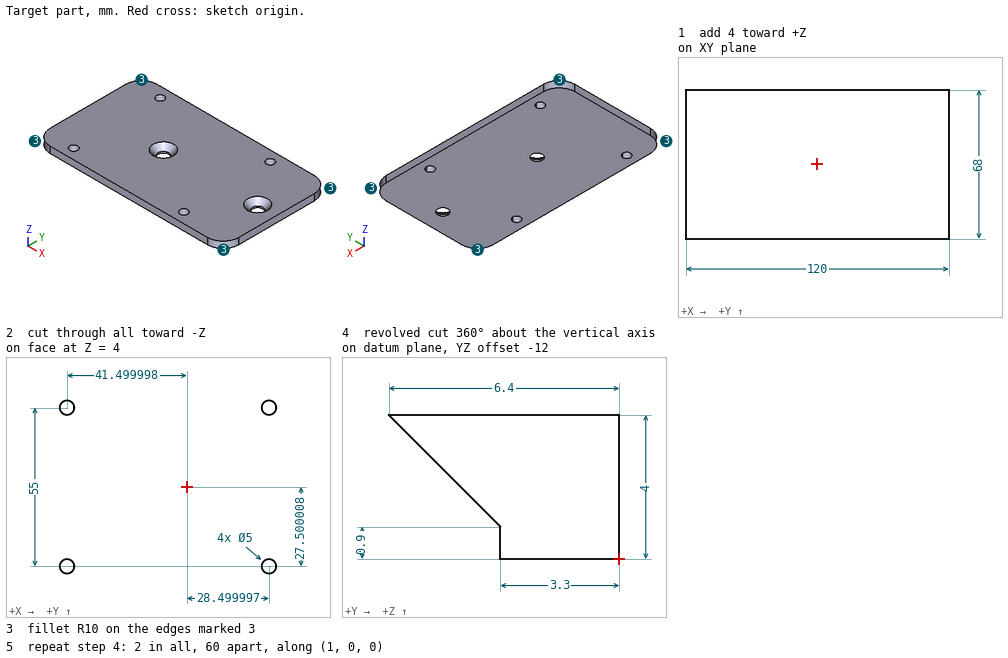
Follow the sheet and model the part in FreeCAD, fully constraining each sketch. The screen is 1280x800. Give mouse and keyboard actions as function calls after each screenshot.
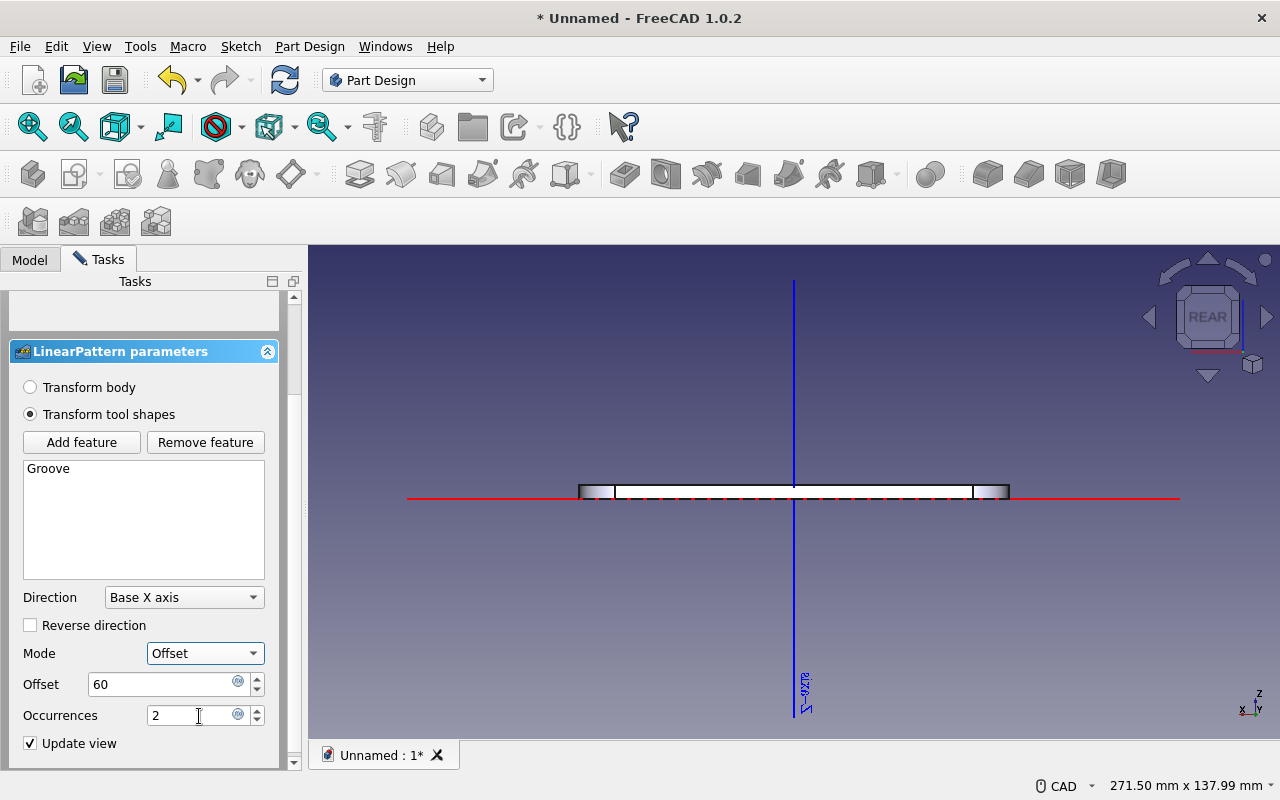
scroll(294, 530, up, 3)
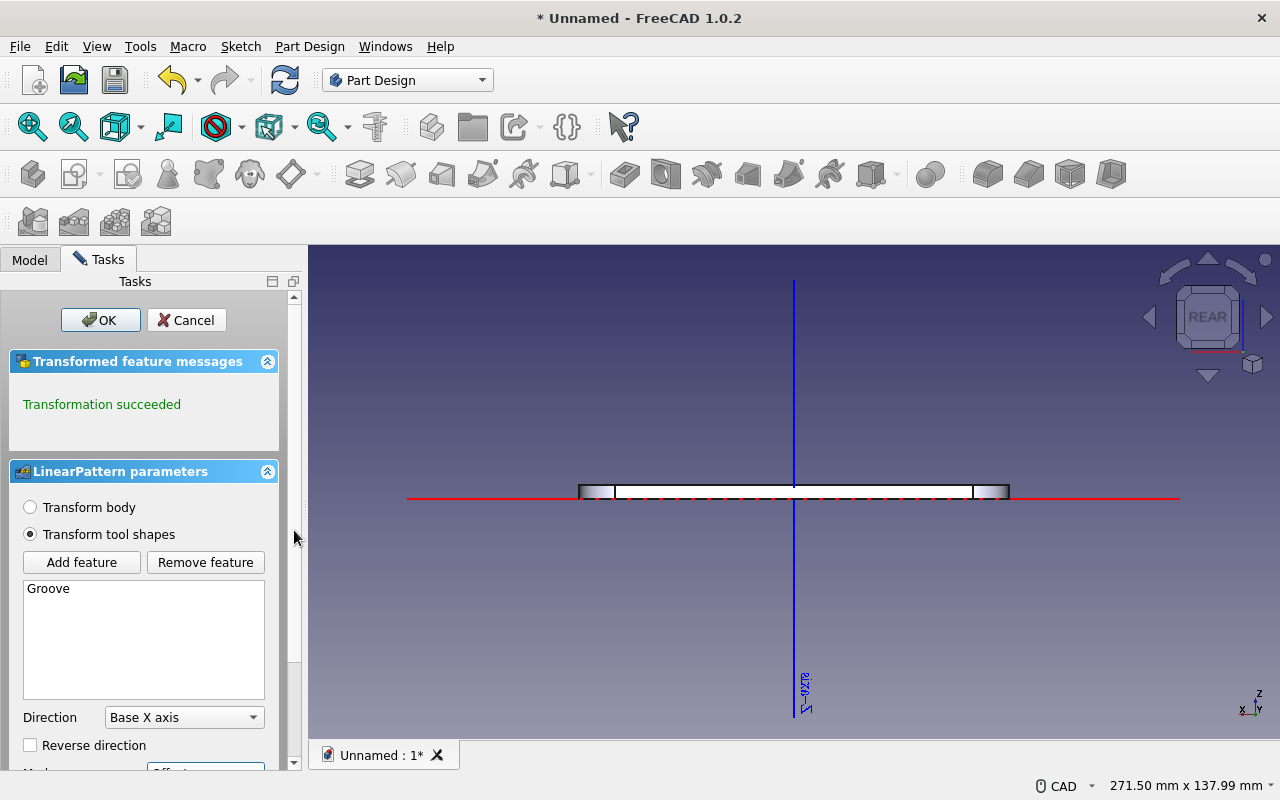
click(101, 320)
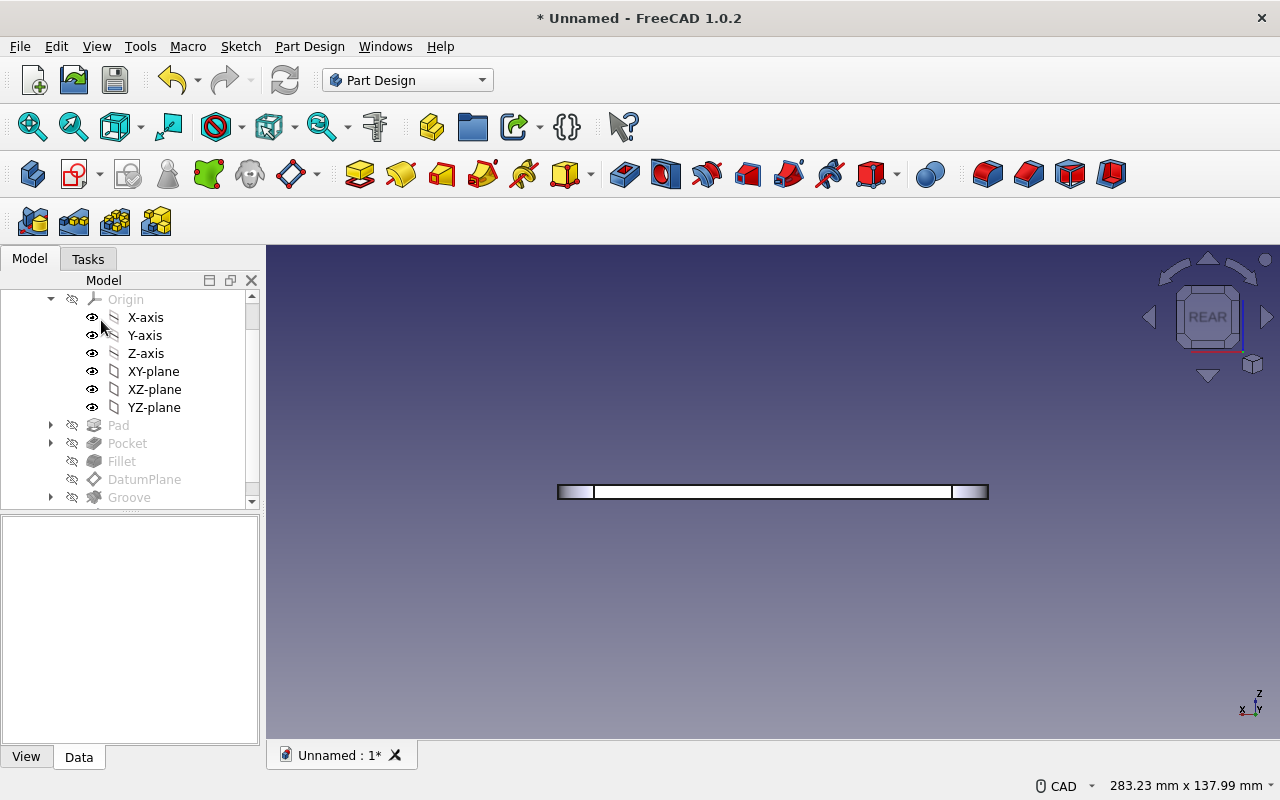
key(0)